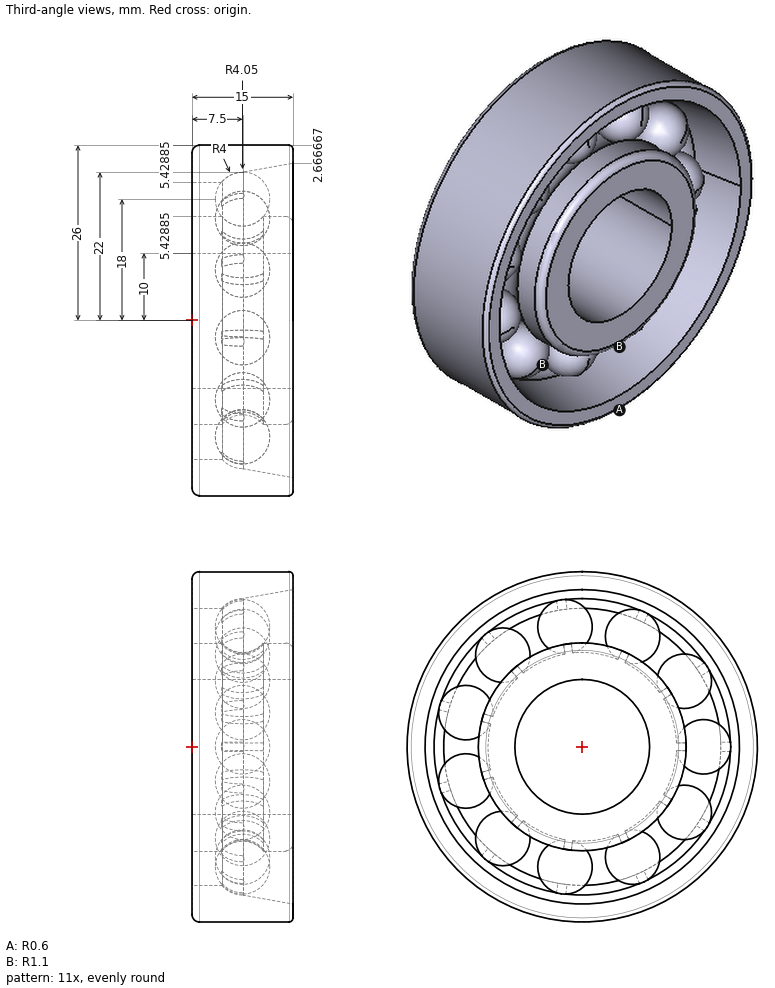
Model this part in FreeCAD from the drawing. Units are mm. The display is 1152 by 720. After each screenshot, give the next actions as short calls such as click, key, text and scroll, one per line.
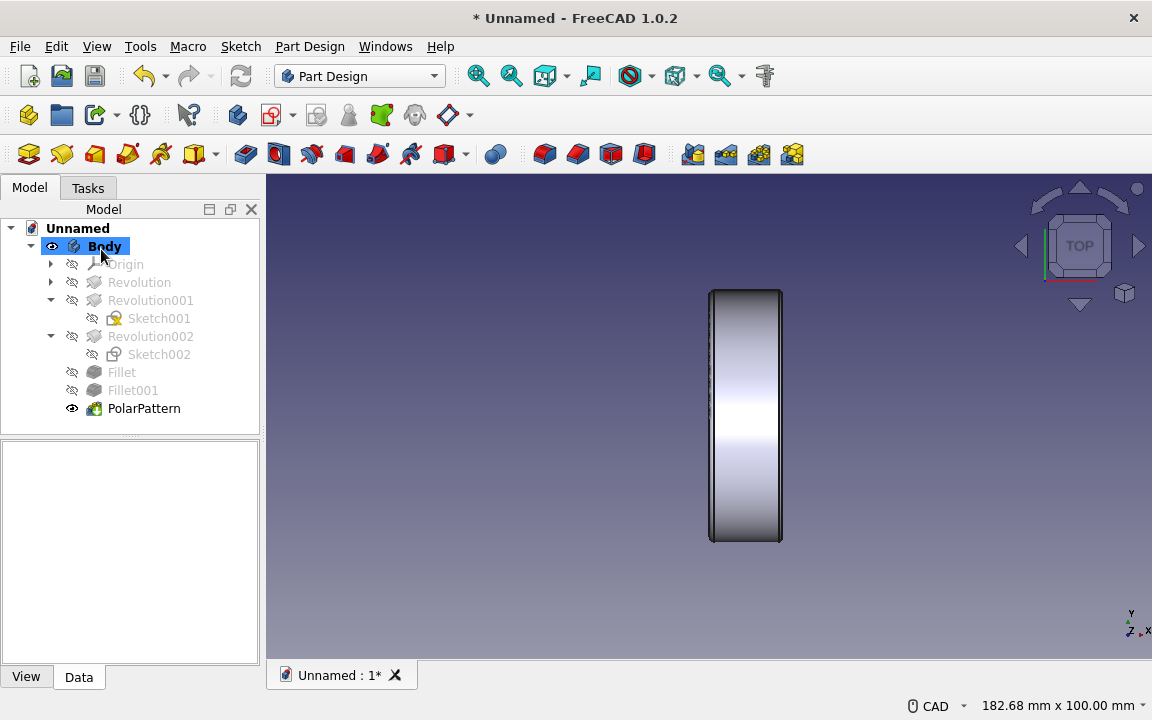
key(0)